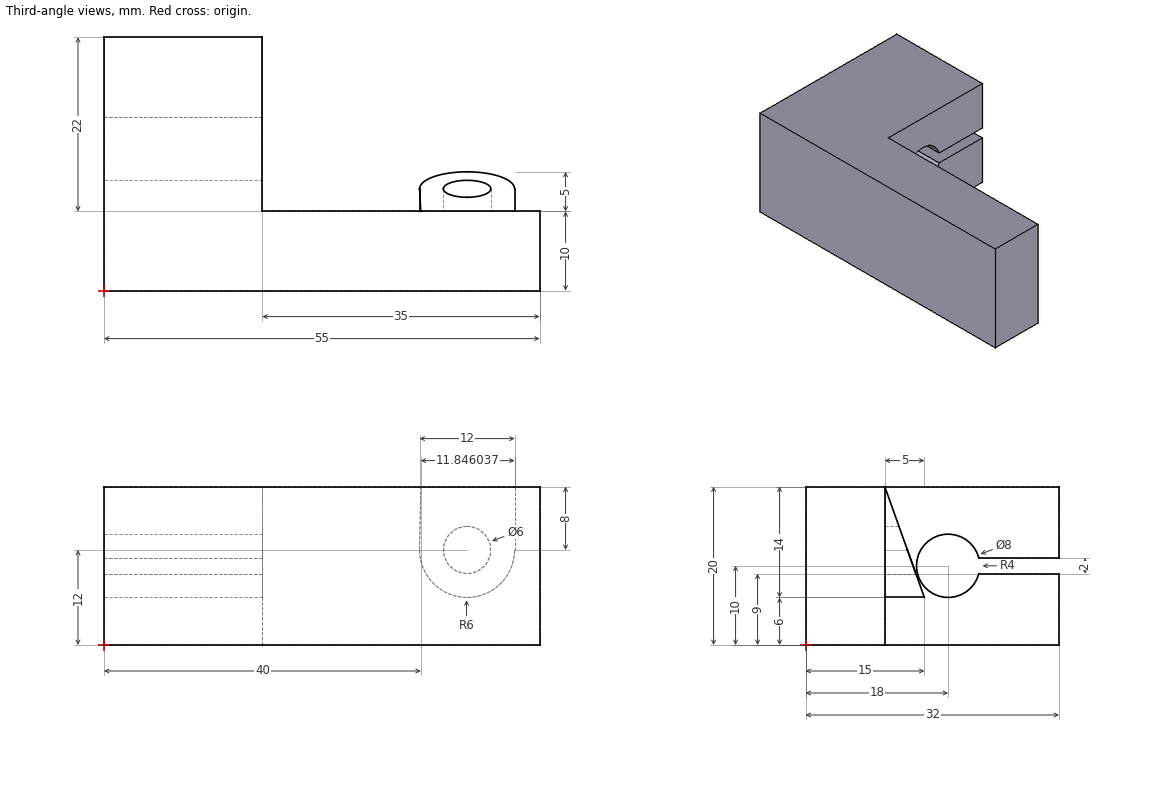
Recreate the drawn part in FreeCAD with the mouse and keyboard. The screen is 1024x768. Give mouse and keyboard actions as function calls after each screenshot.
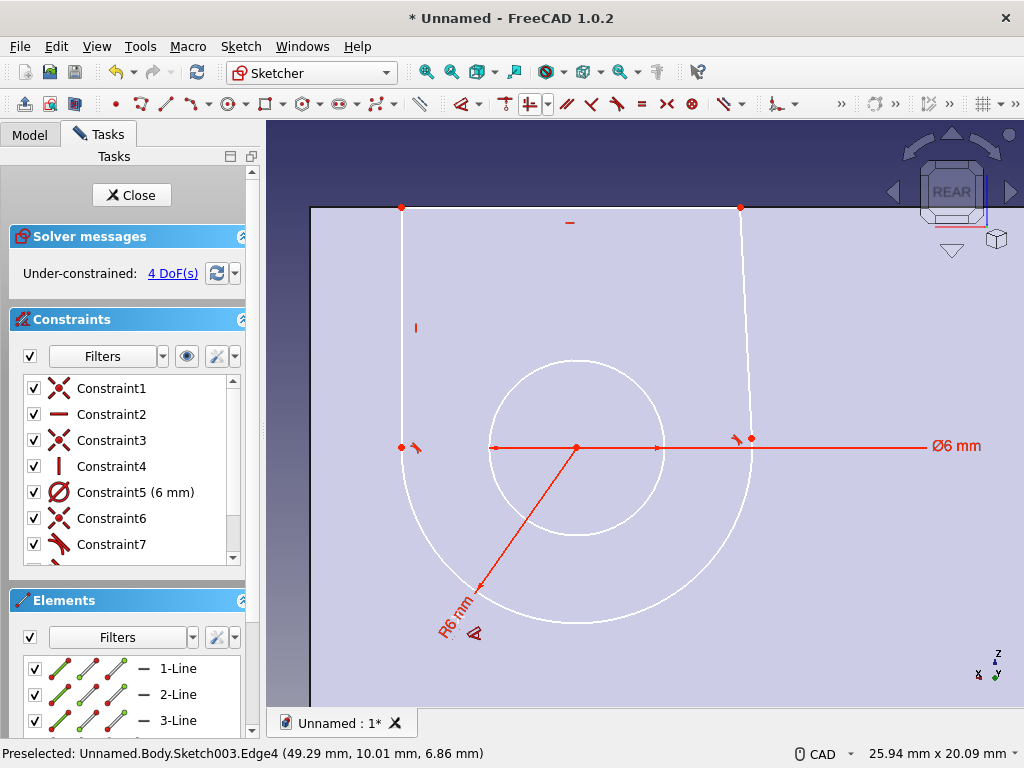
click(402, 280)
click(368, 328)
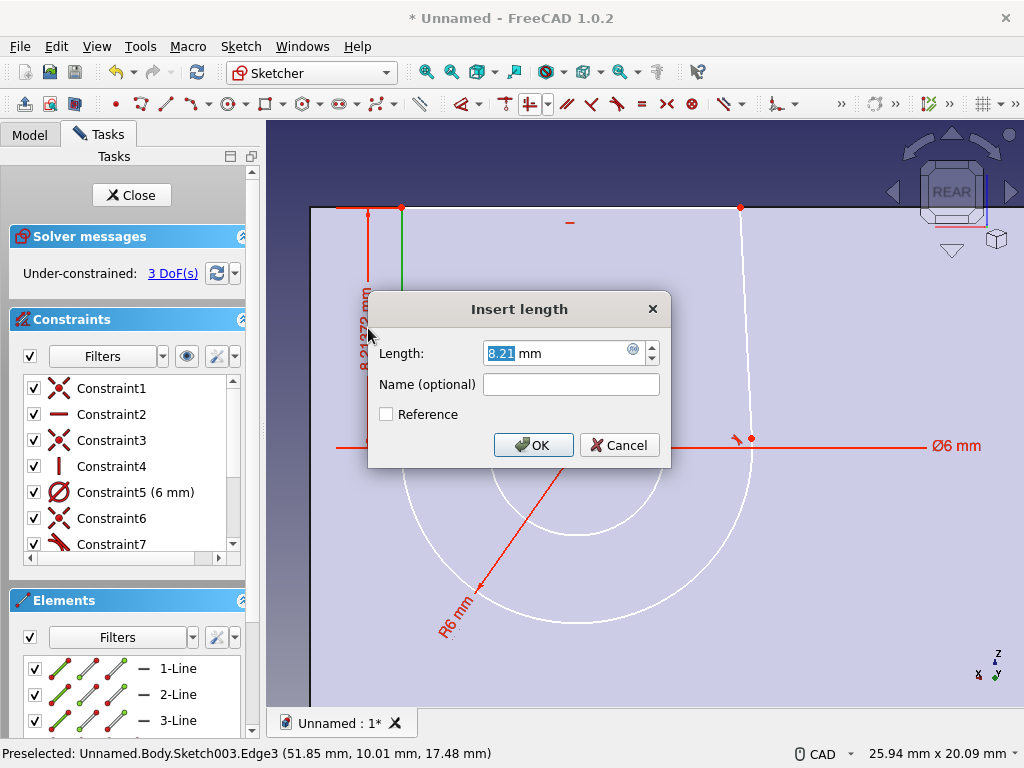
text(8)
key(Return)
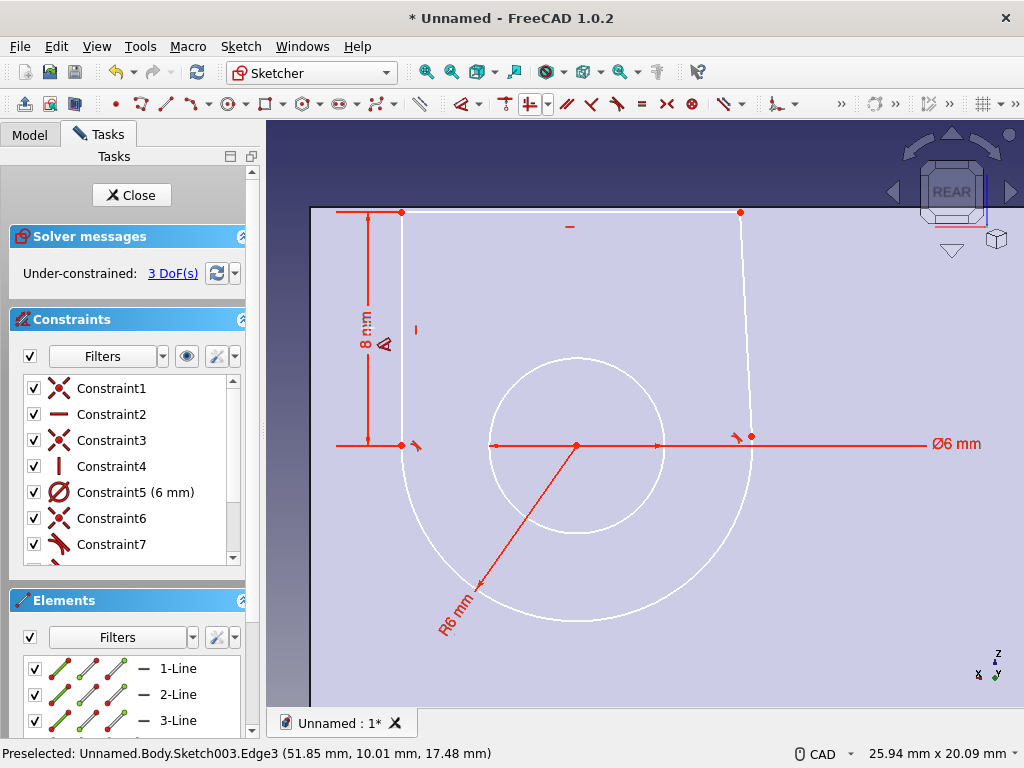
click(577, 446)
click(543, 562)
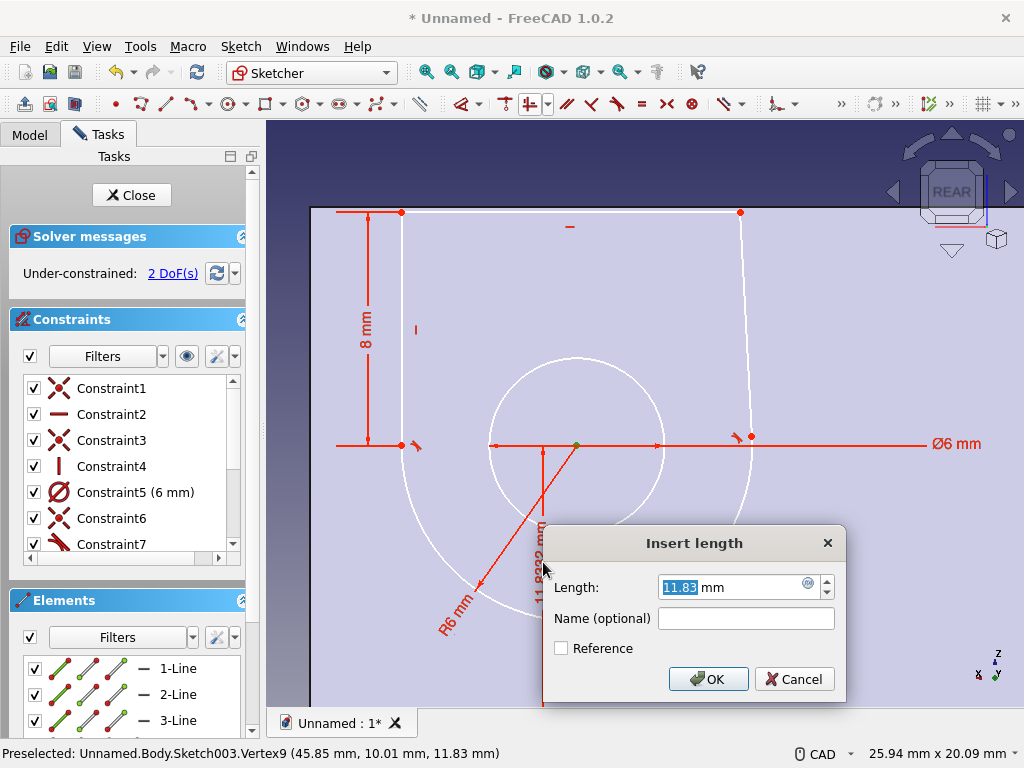
text(12)
key(Return)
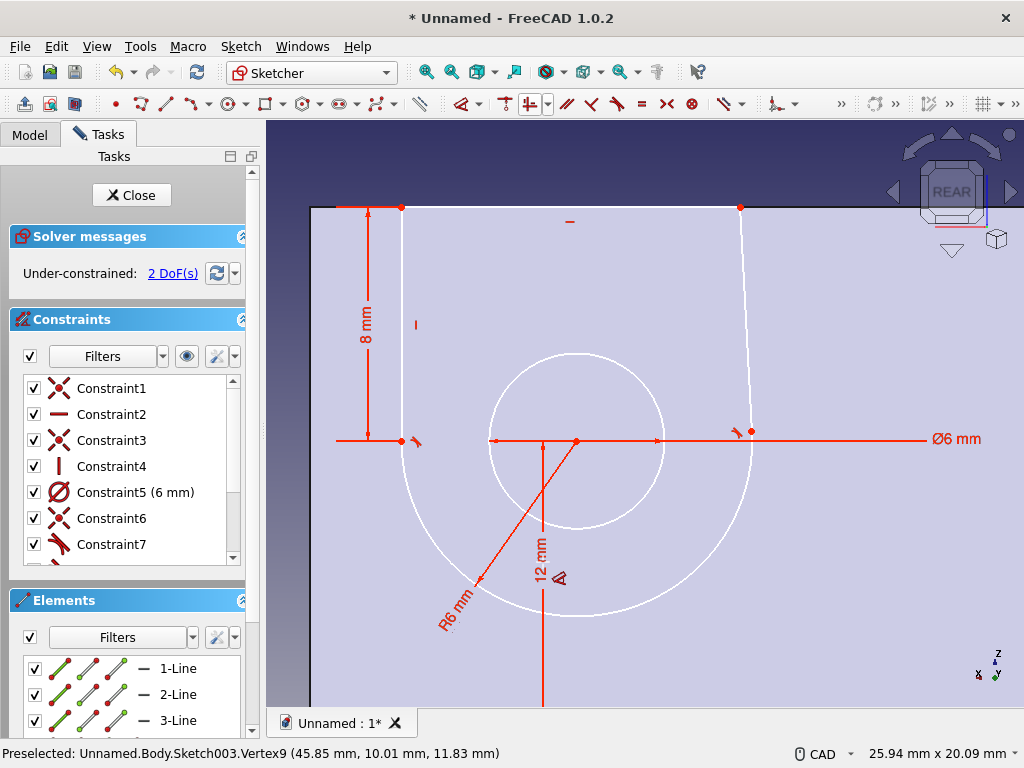
click(740, 207)
click(800, 173)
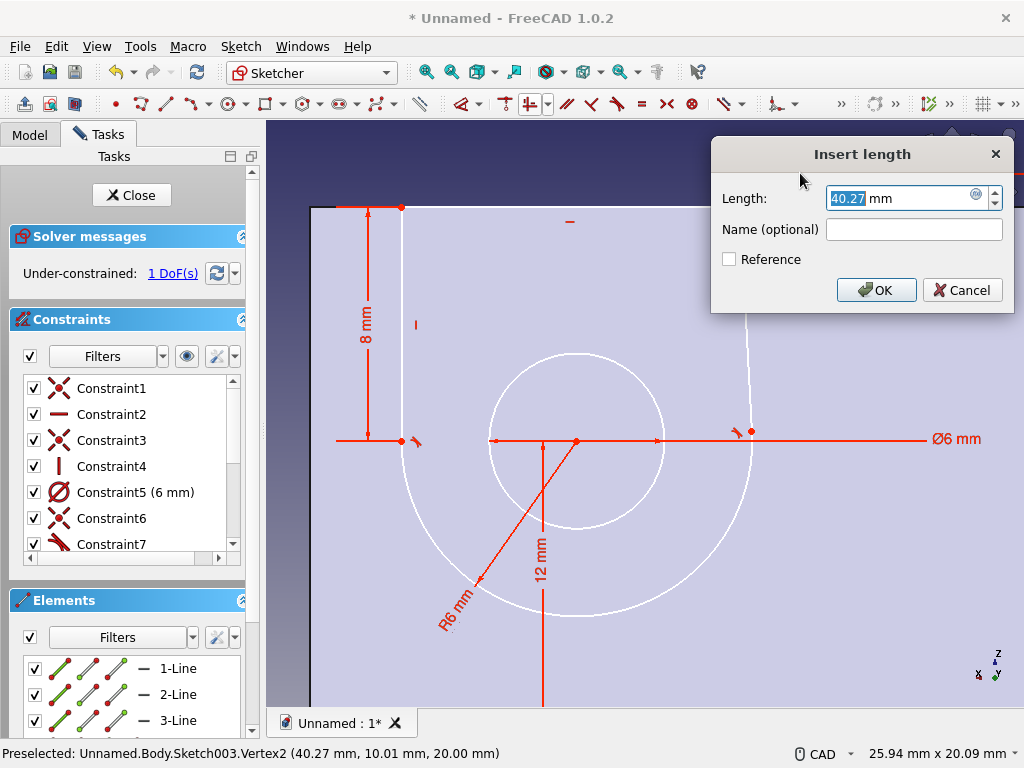
text(40)
key(Return)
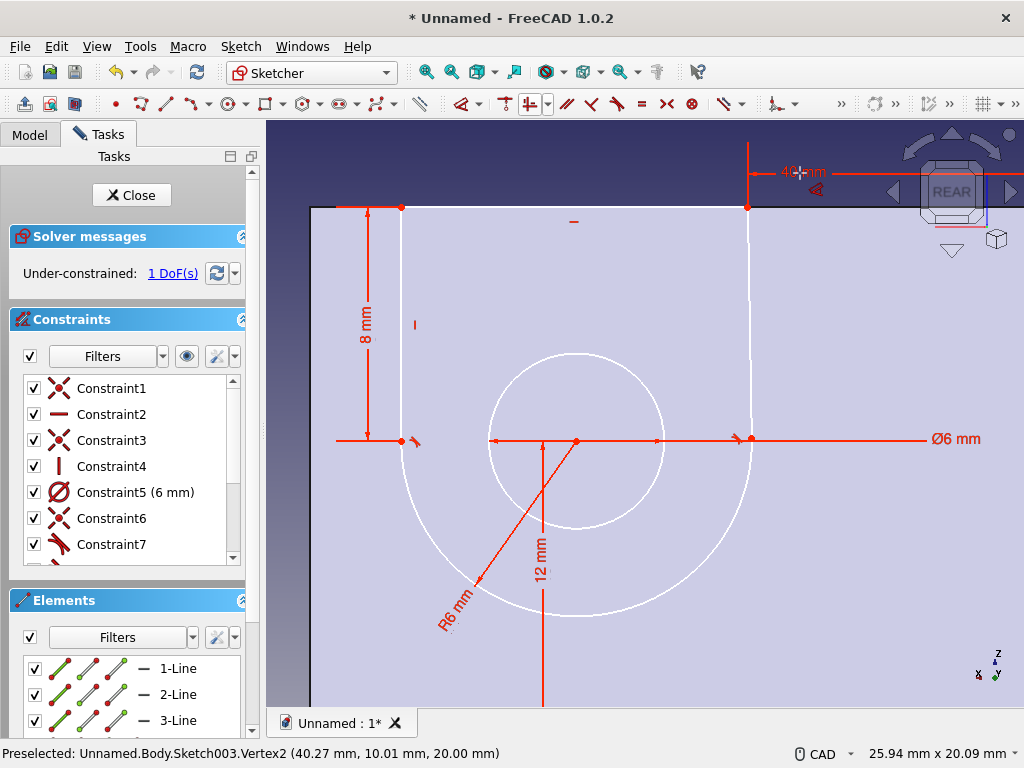
click(644, 207)
click(575, 173)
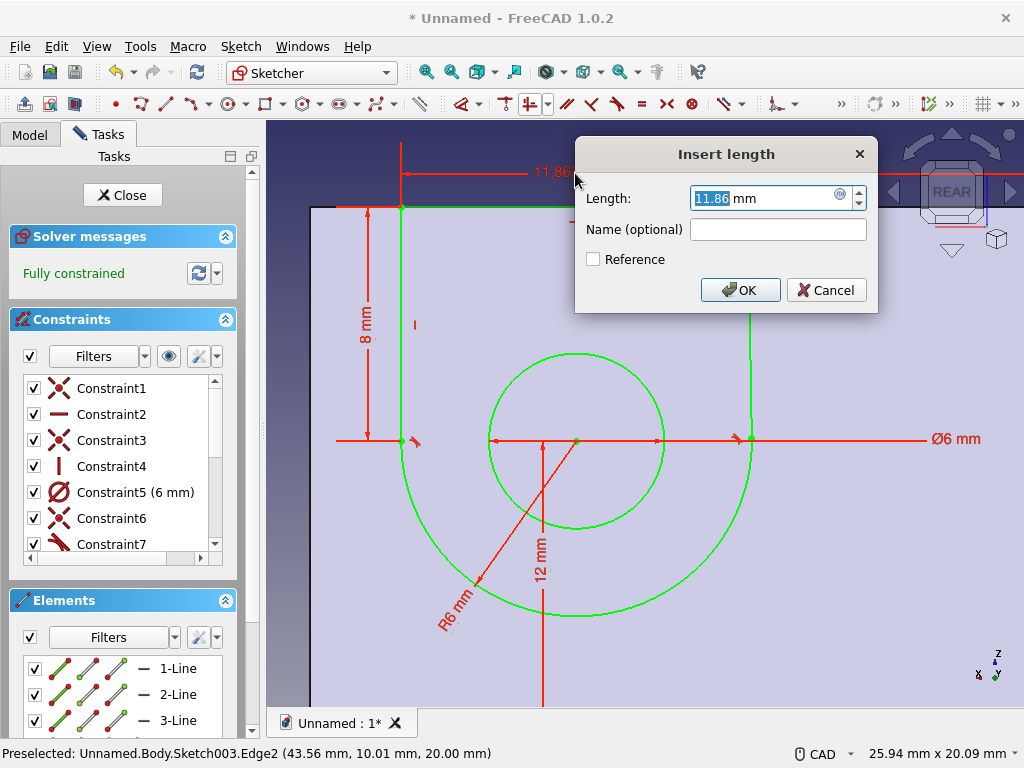
text(11.846037)
key(Return)
key(Escape)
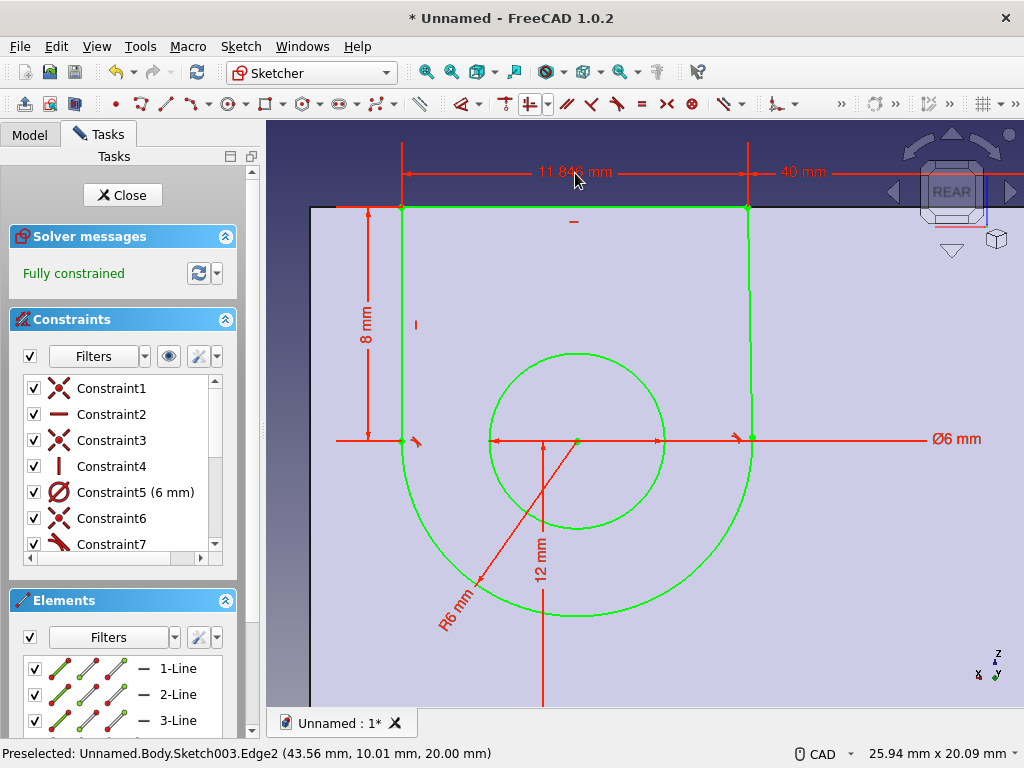
click(123, 195)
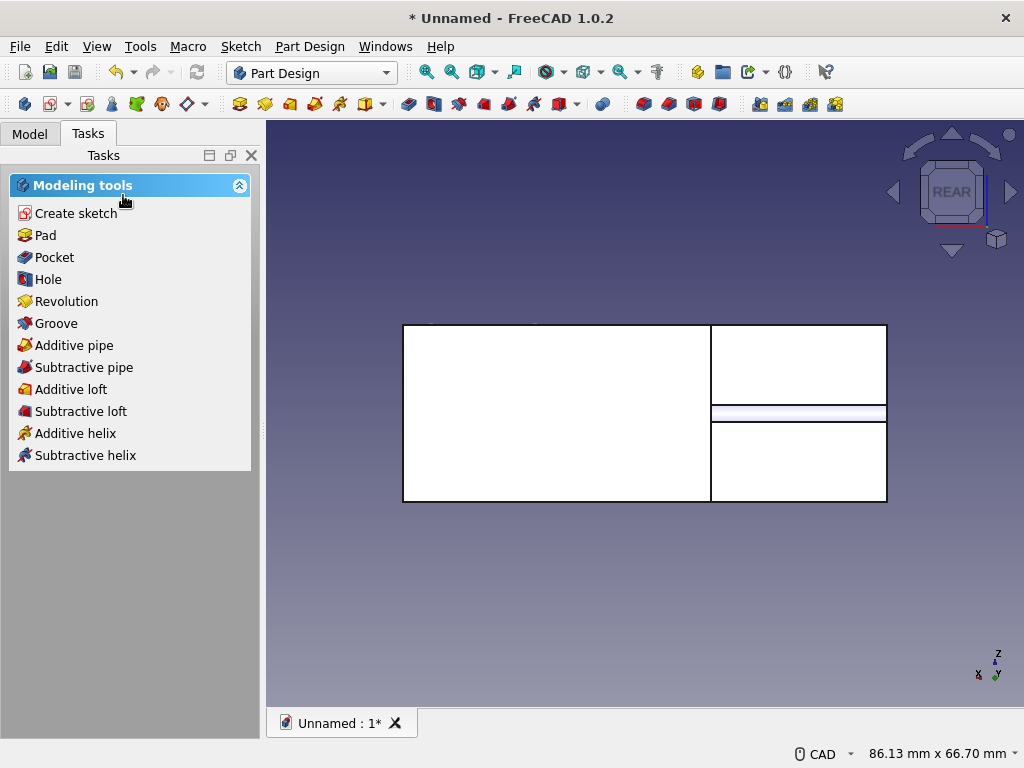
click(240, 104)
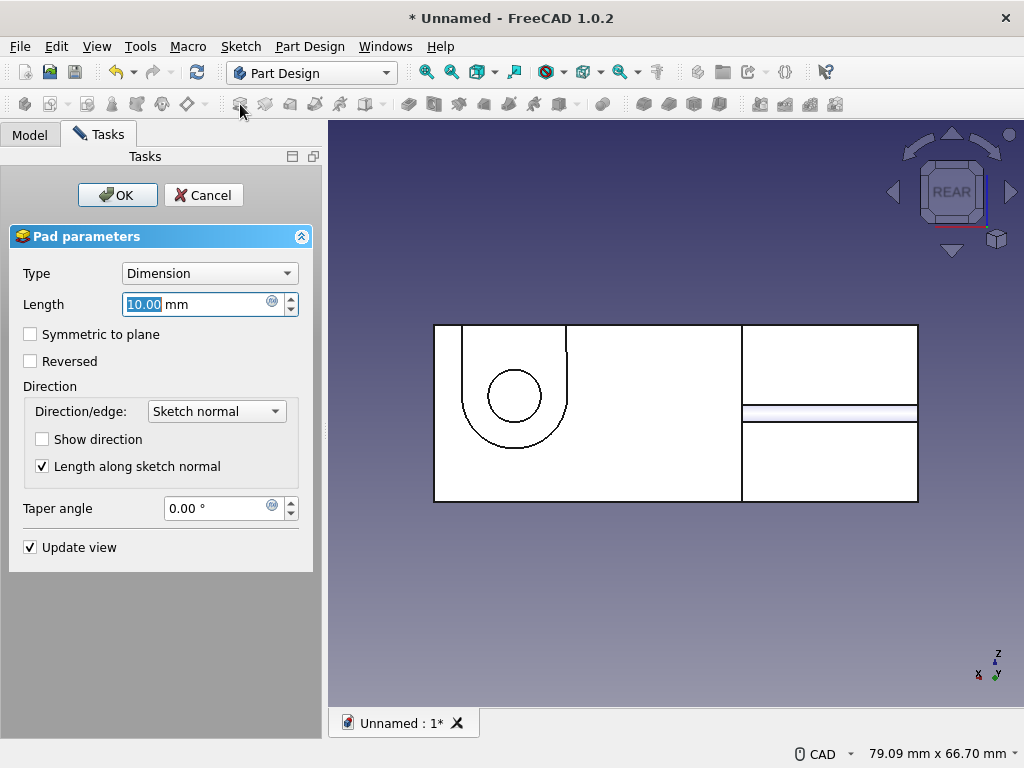
text(5)
key(Tab)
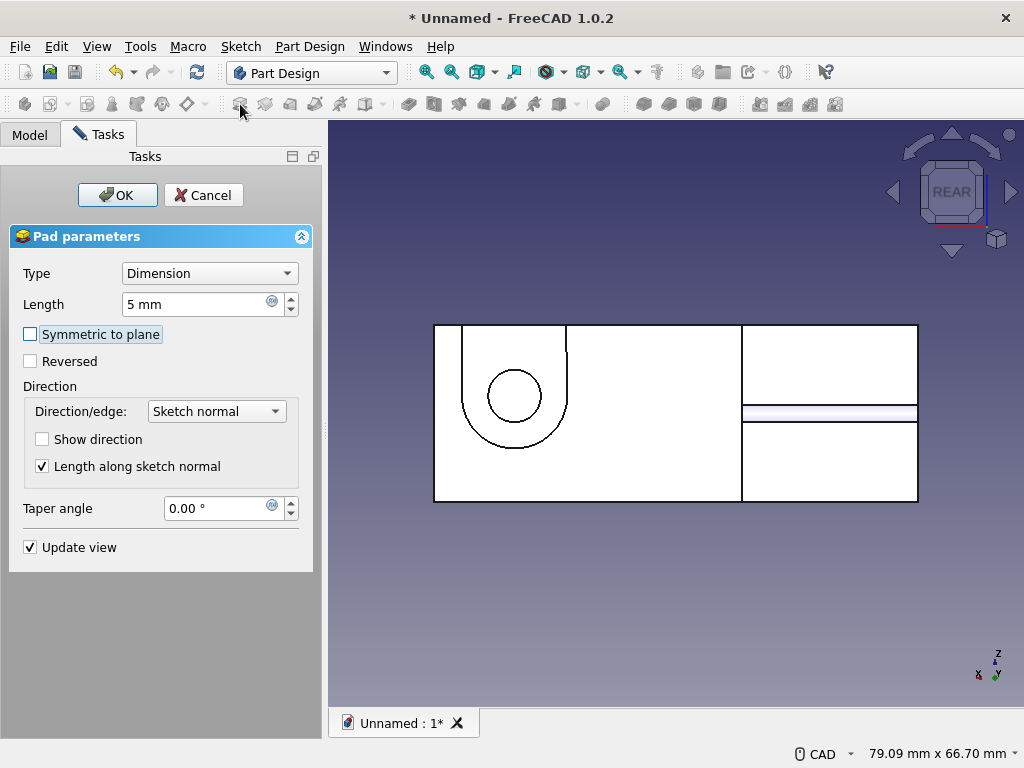
click(118, 195)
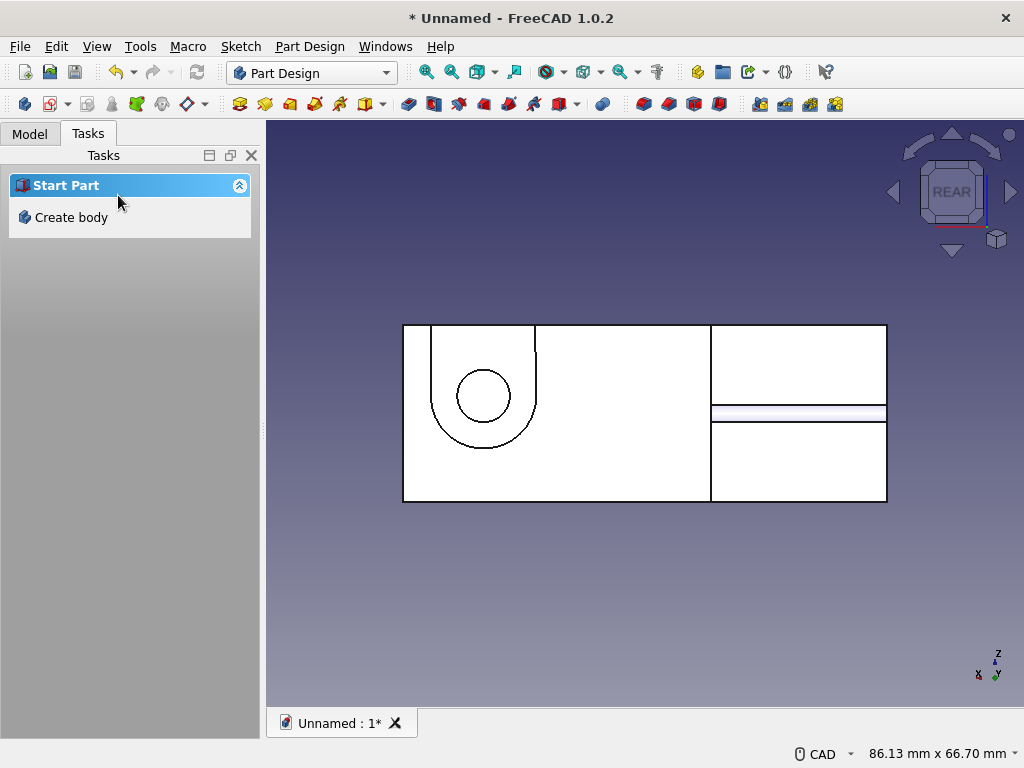
key(0)